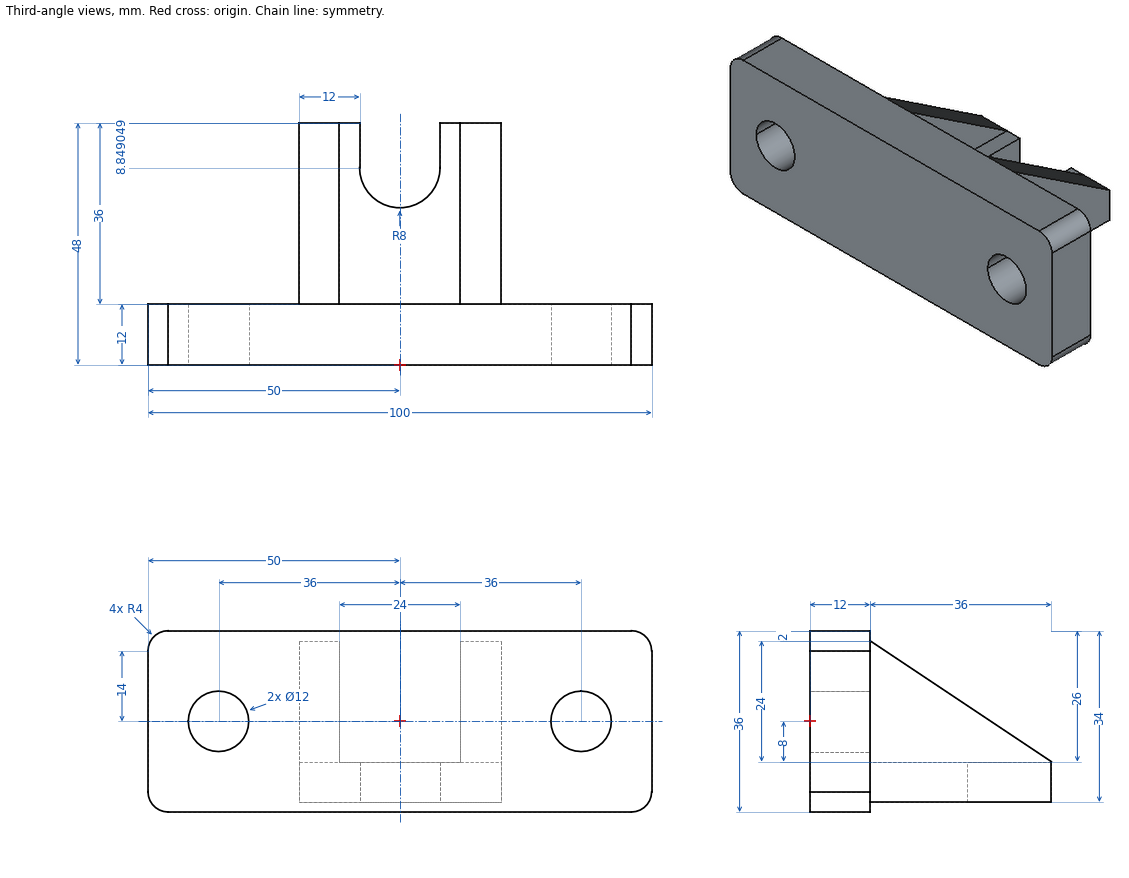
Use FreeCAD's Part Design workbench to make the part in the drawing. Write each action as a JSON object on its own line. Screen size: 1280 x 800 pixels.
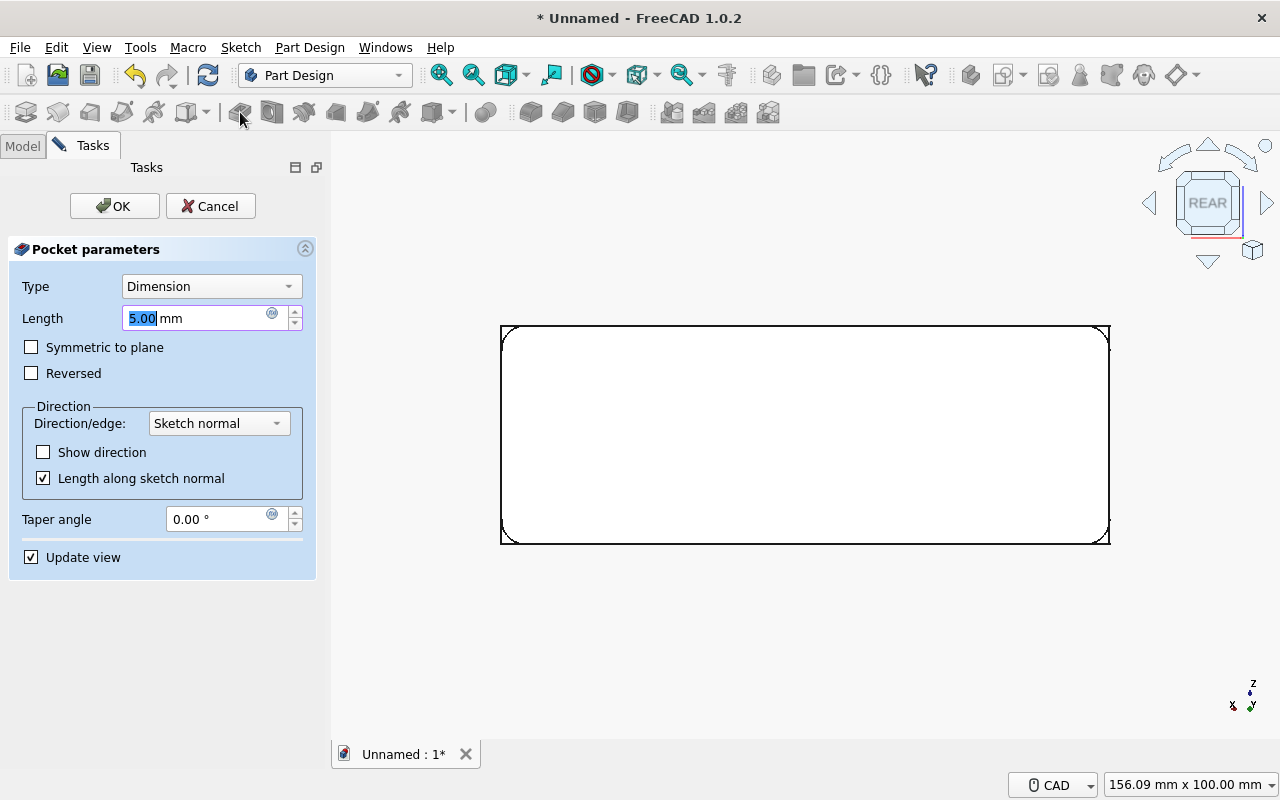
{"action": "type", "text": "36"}
{"action": "key", "text": "Tab"}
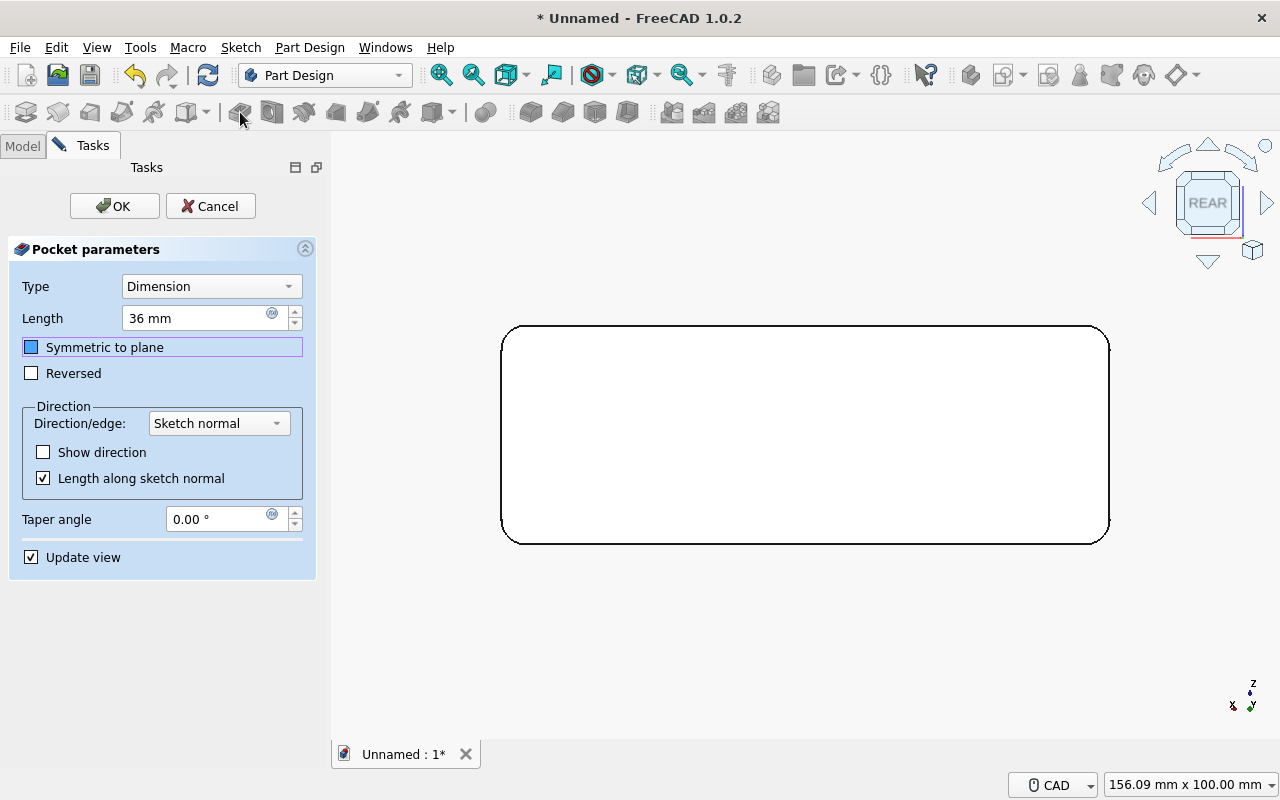
{"action": "left_click", "coordinate": [115, 206]}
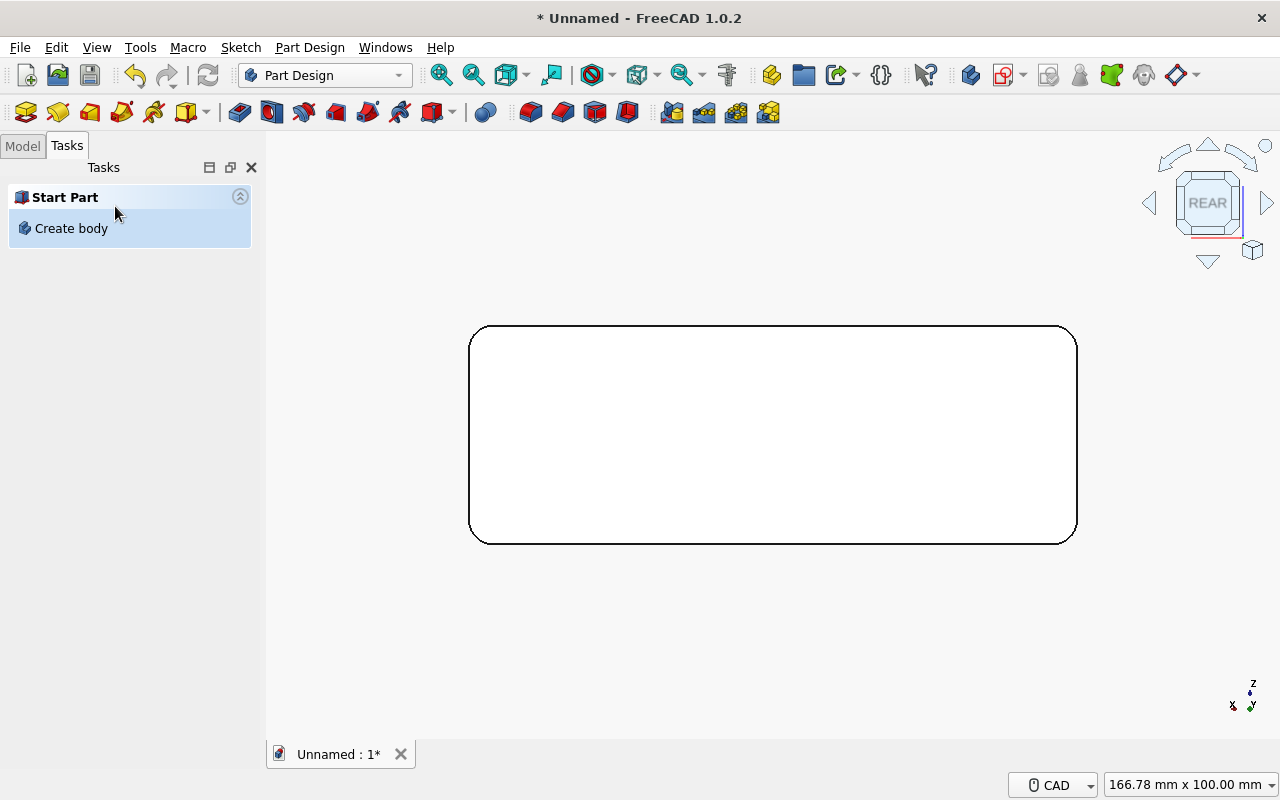
{"action": "left_click", "coordinate": [599, 434]}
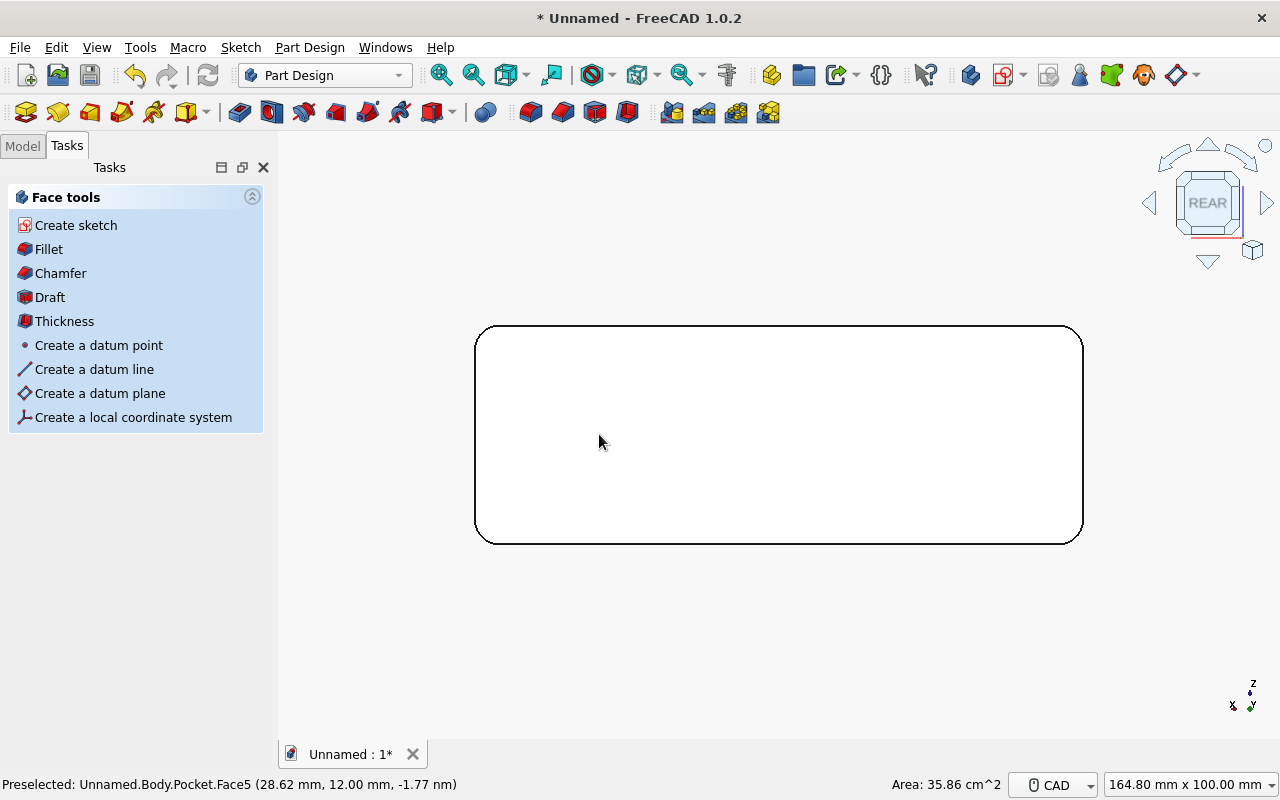
{"action": "left_click", "coordinate": [1004, 76]}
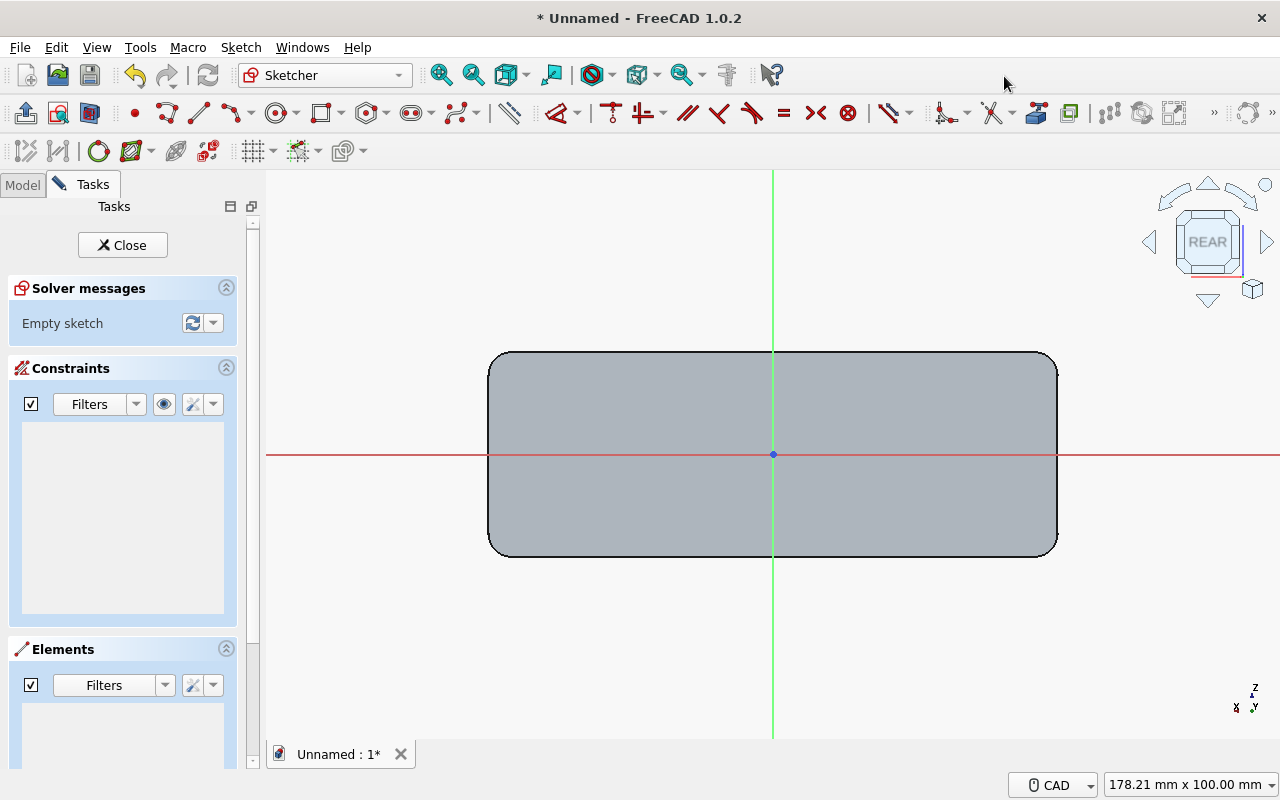
{"action": "left_click", "coordinate": [276, 114]}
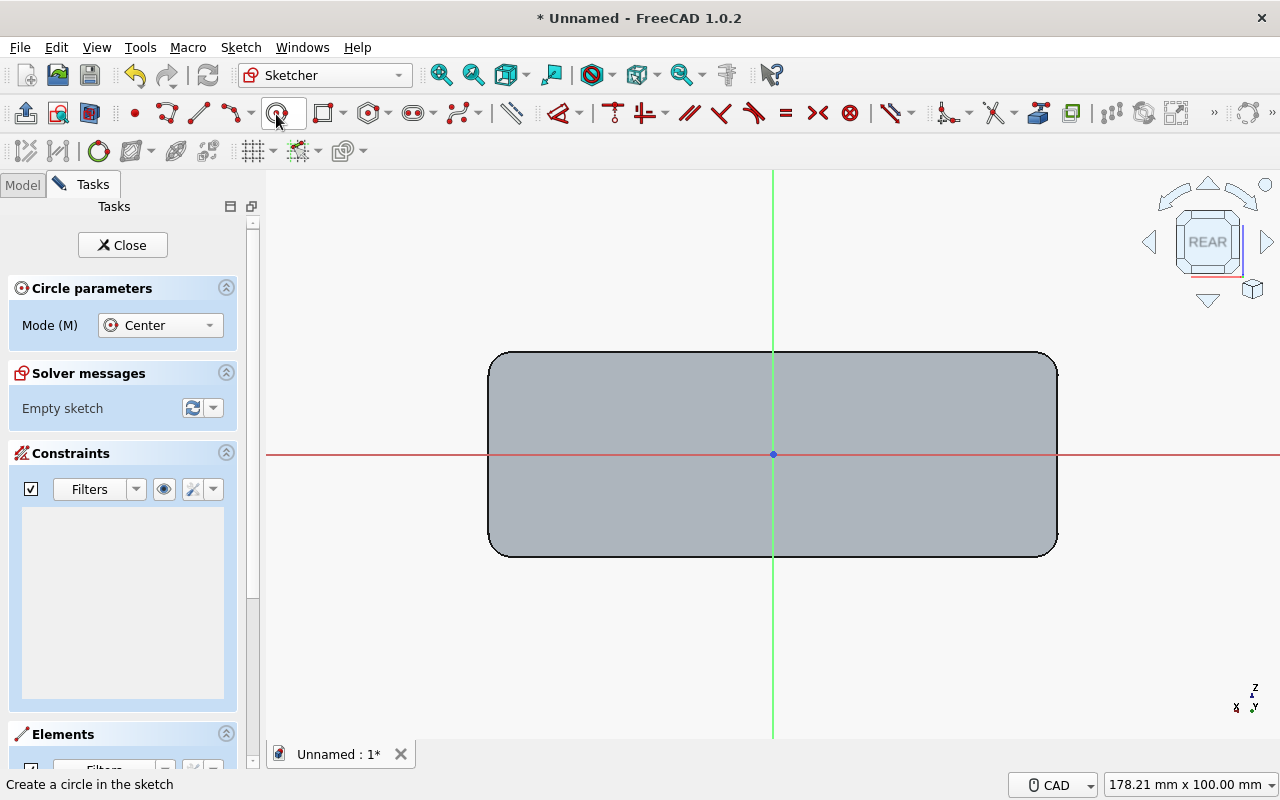
{"action": "left_click", "coordinate": [978, 455]}
{"action": "mouse_move", "coordinate": [1002, 430]}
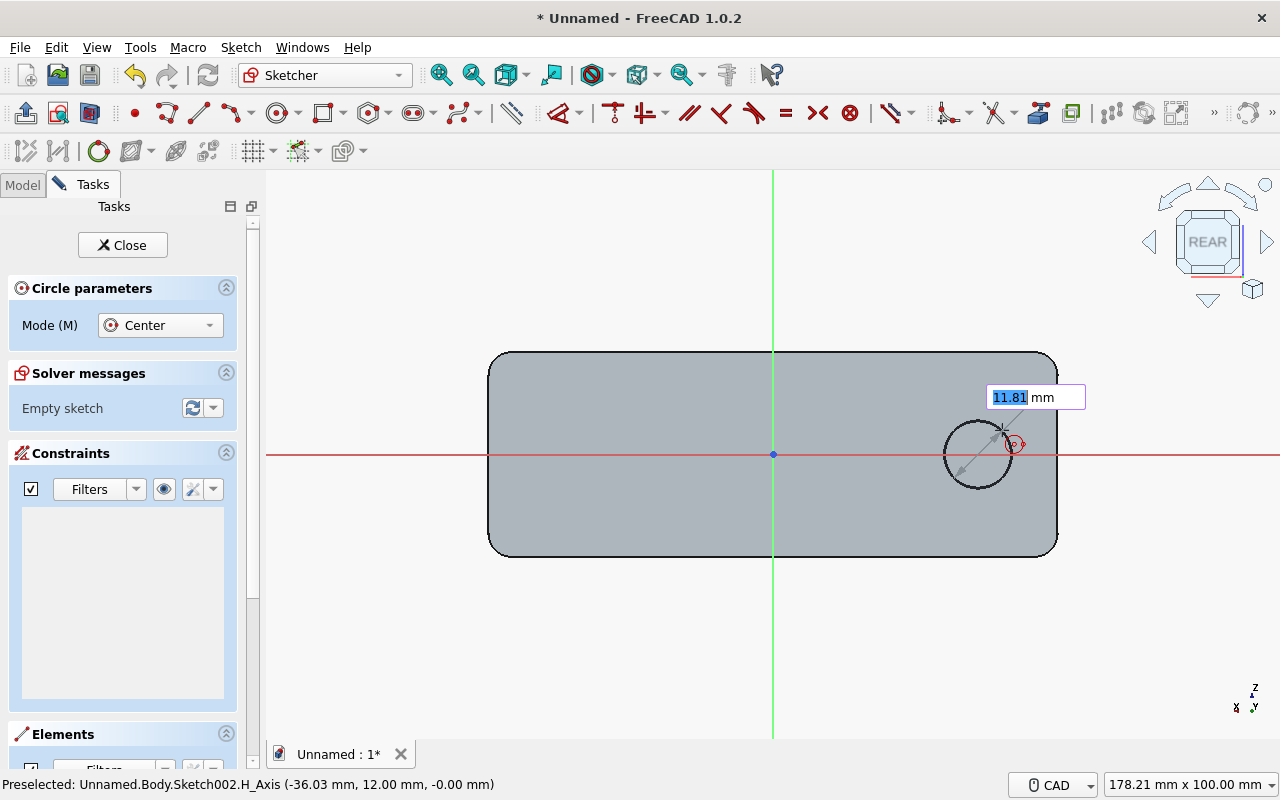
{"action": "type", "text": "12"}
{"action": "key", "text": "Return"}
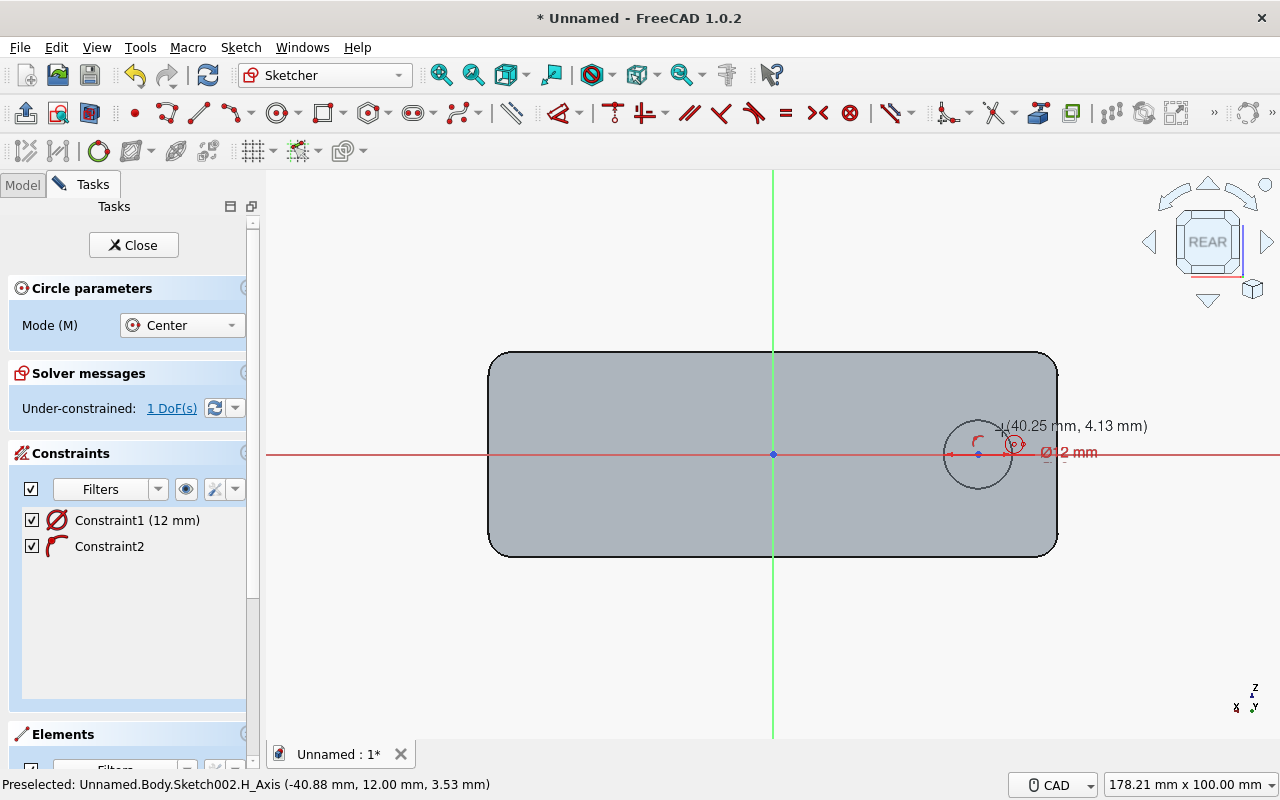
{"action": "left_click", "coordinate": [568, 455]}
{"action": "mouse_move", "coordinate": [592, 430]}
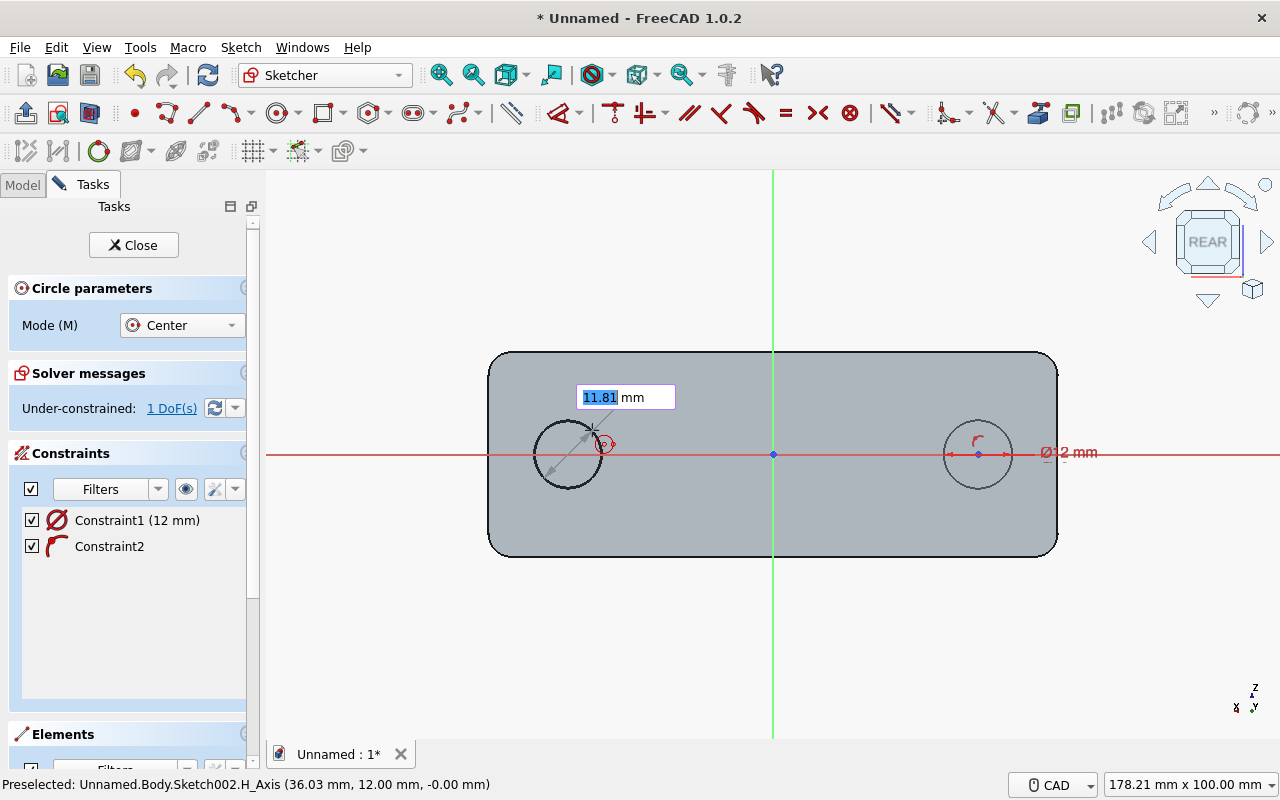
{"action": "type", "text": "12"}
{"action": "key", "text": "Return"}
{"action": "key", "text": "Escape"}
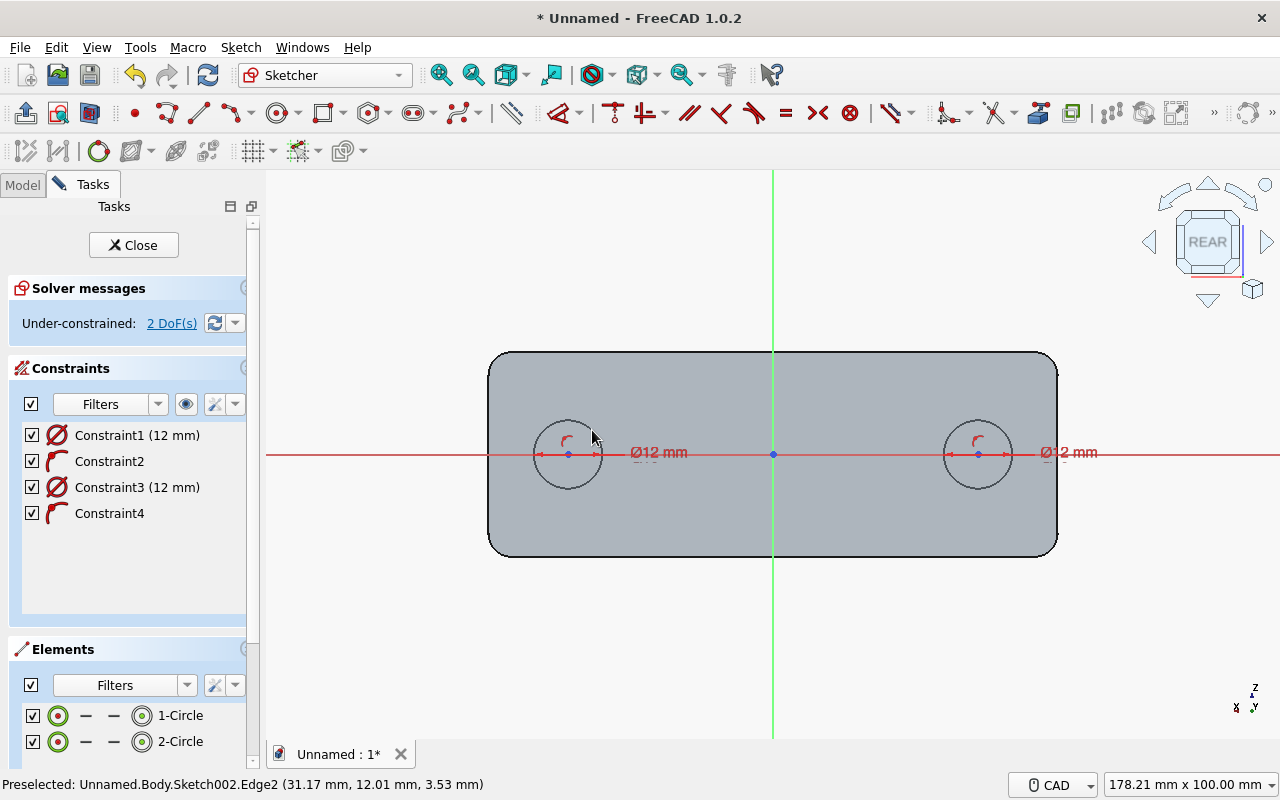
{"action": "left_click", "coordinate": [558, 114]}